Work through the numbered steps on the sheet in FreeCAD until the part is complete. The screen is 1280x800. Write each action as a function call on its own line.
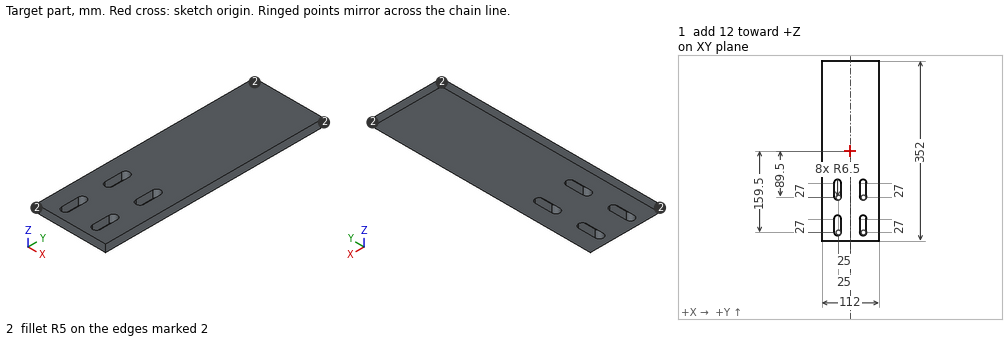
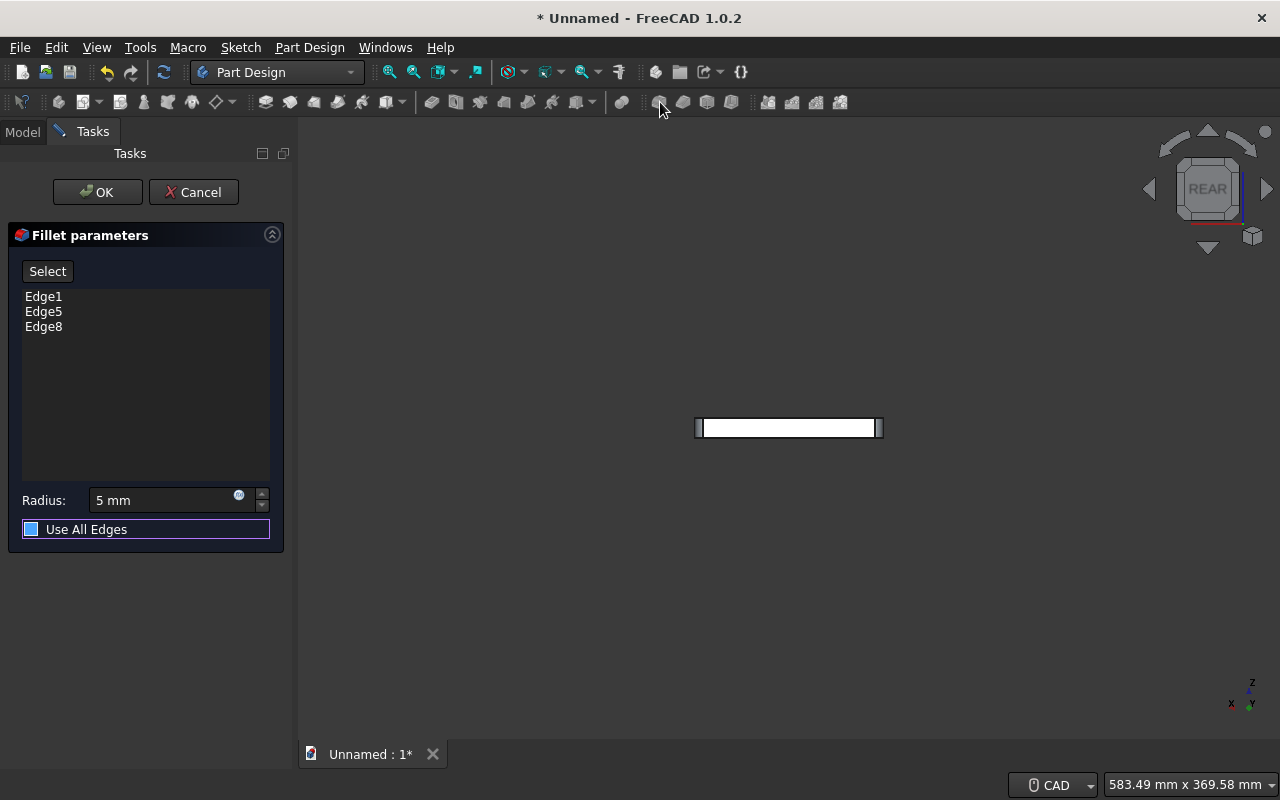
click(98, 192)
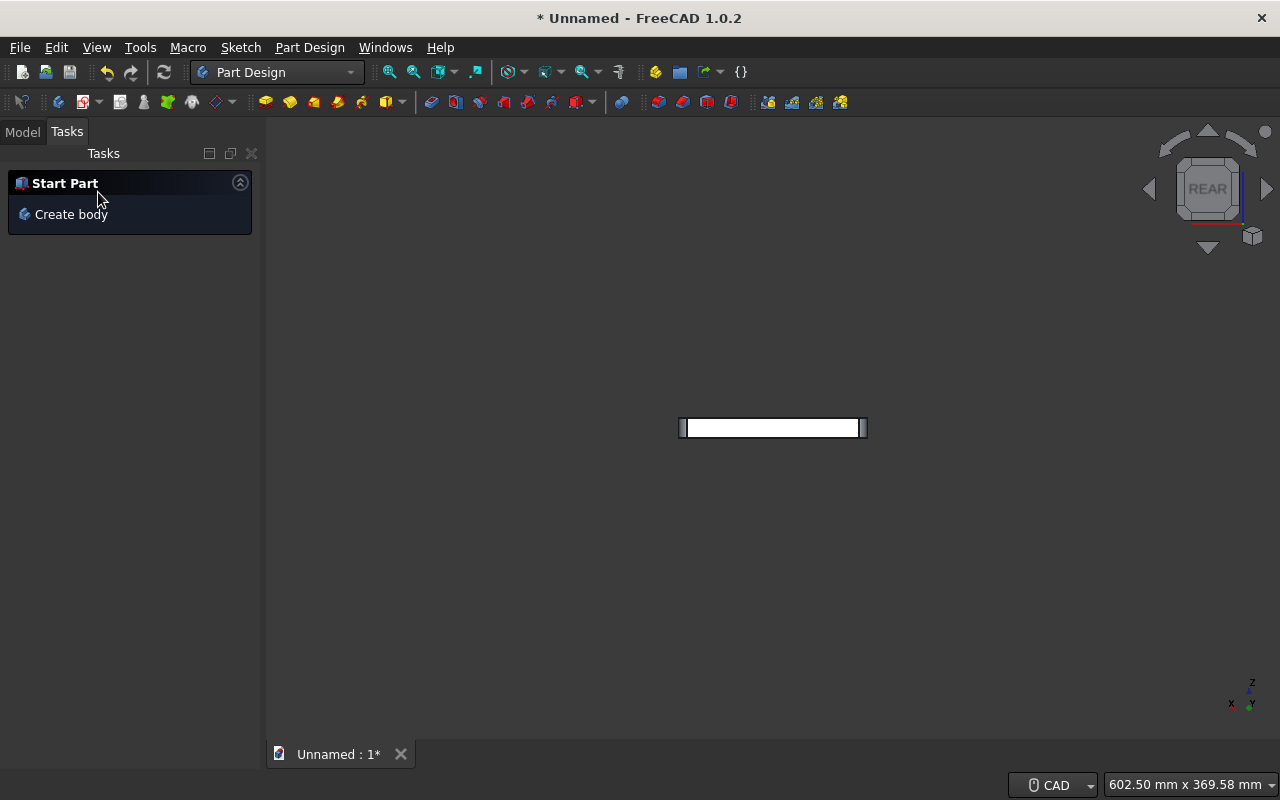
key(0)